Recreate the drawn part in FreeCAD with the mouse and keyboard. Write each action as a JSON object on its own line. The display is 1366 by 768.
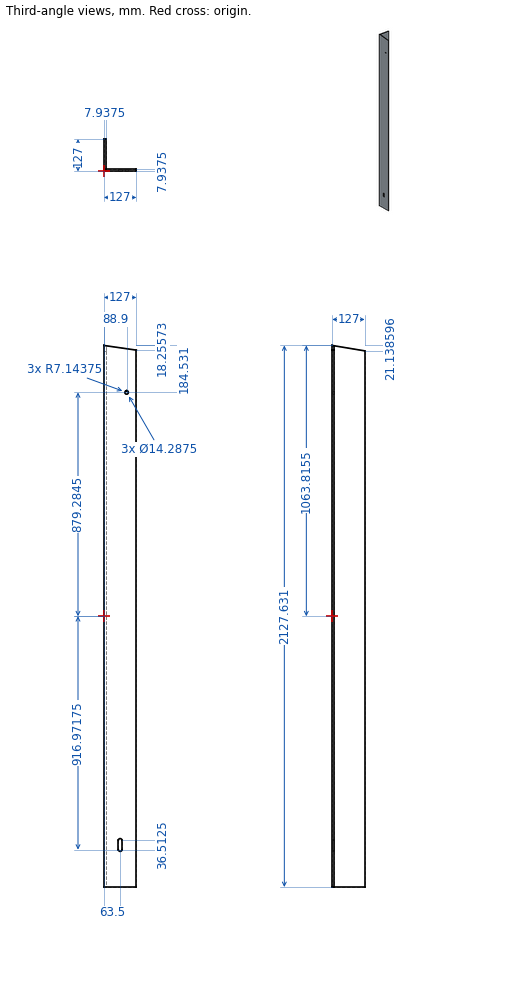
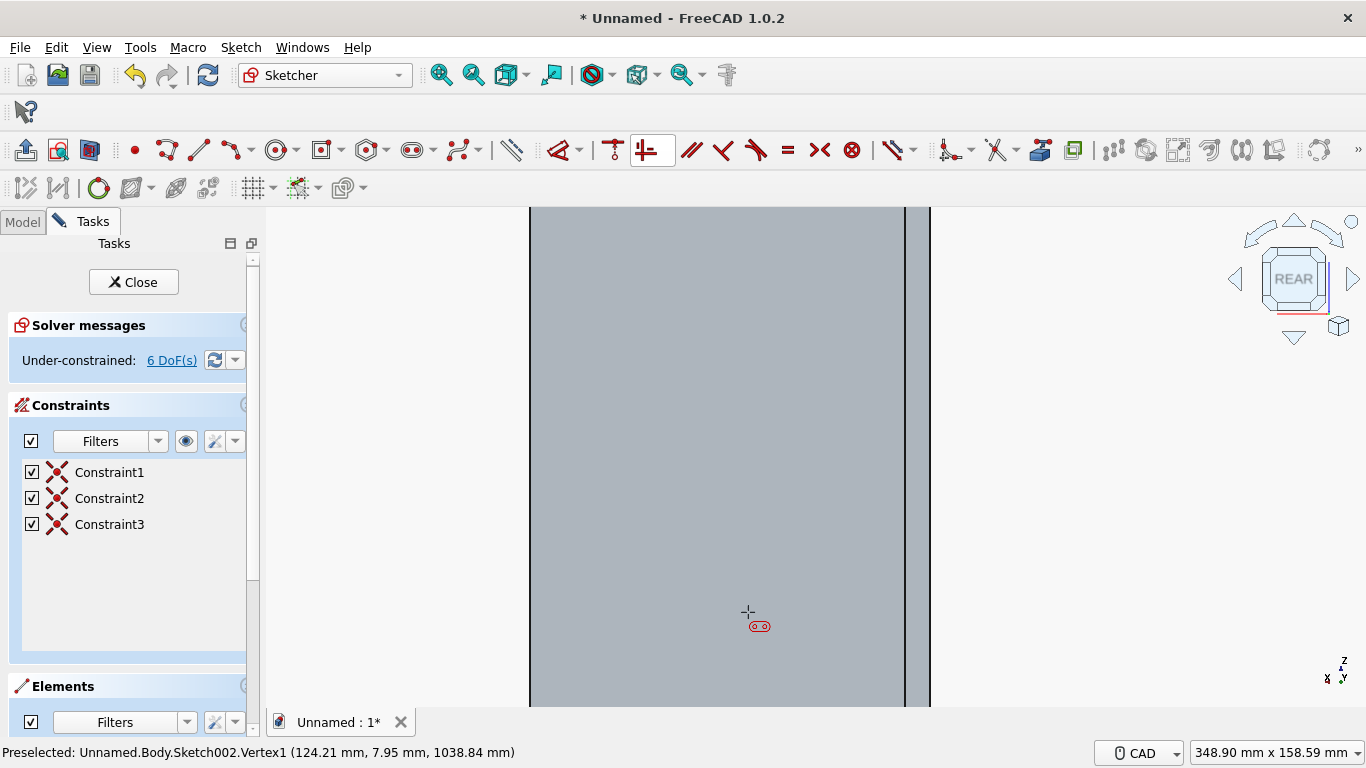
{"action": "scroll", "coordinate": [749, 649], "scroll_direction": "down", "scroll_amount": 15}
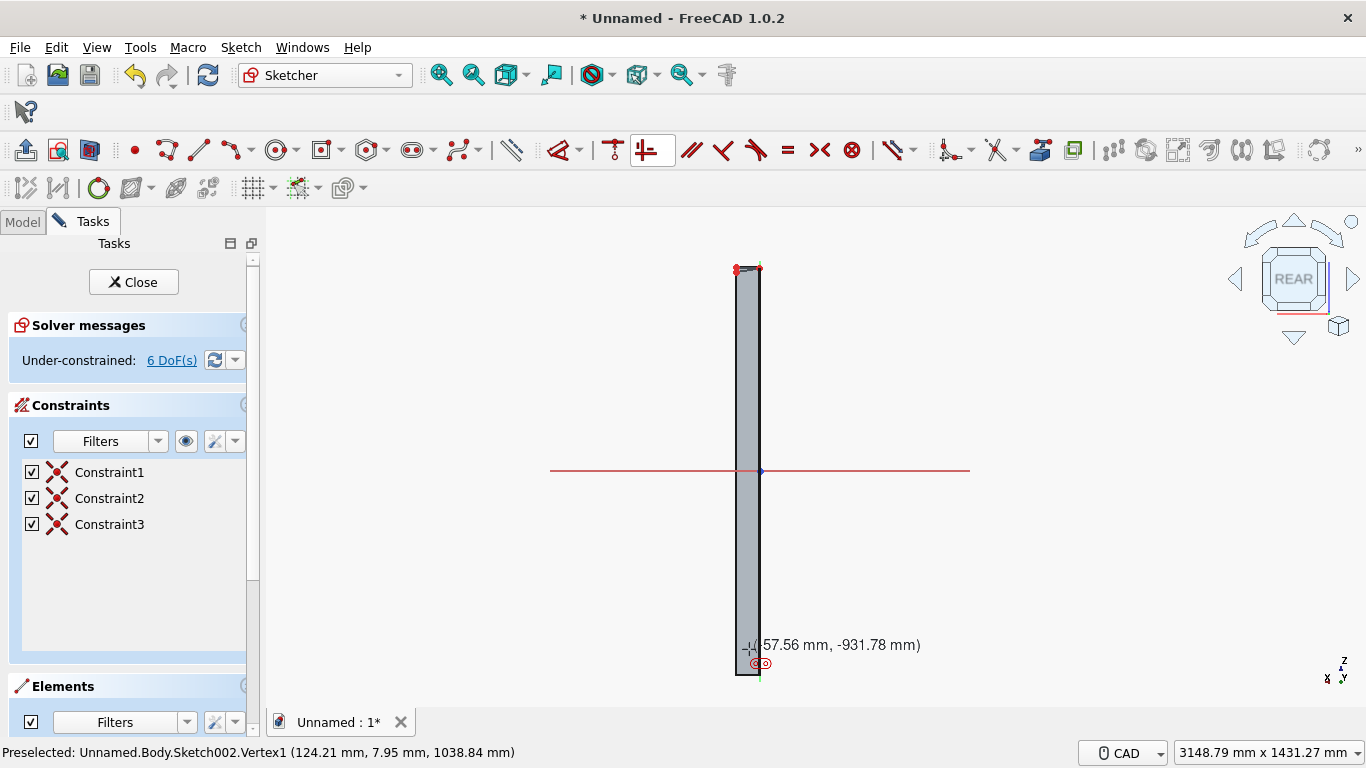
{"action": "scroll", "coordinate": [748, 647], "scroll_direction": "up", "scroll_amount": 2}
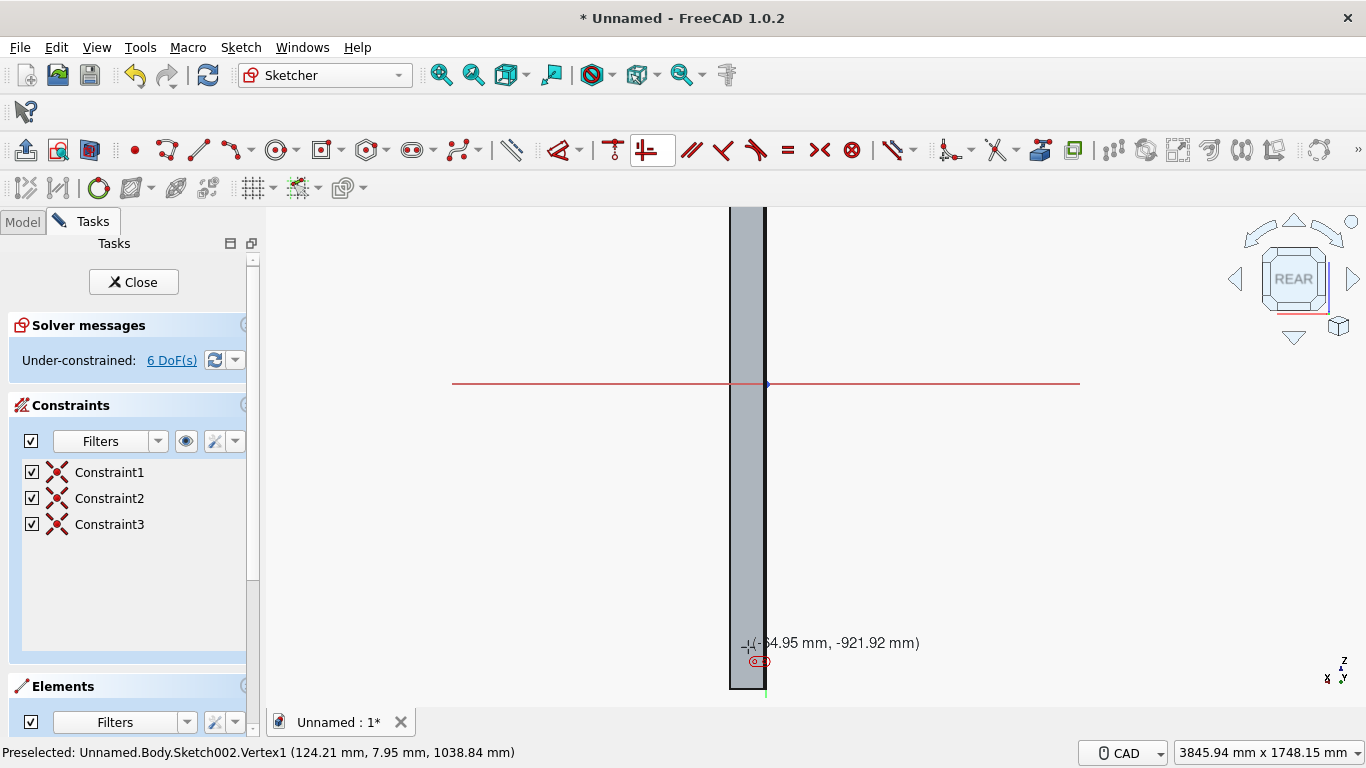
{"action": "left_click", "coordinate": [748, 647]}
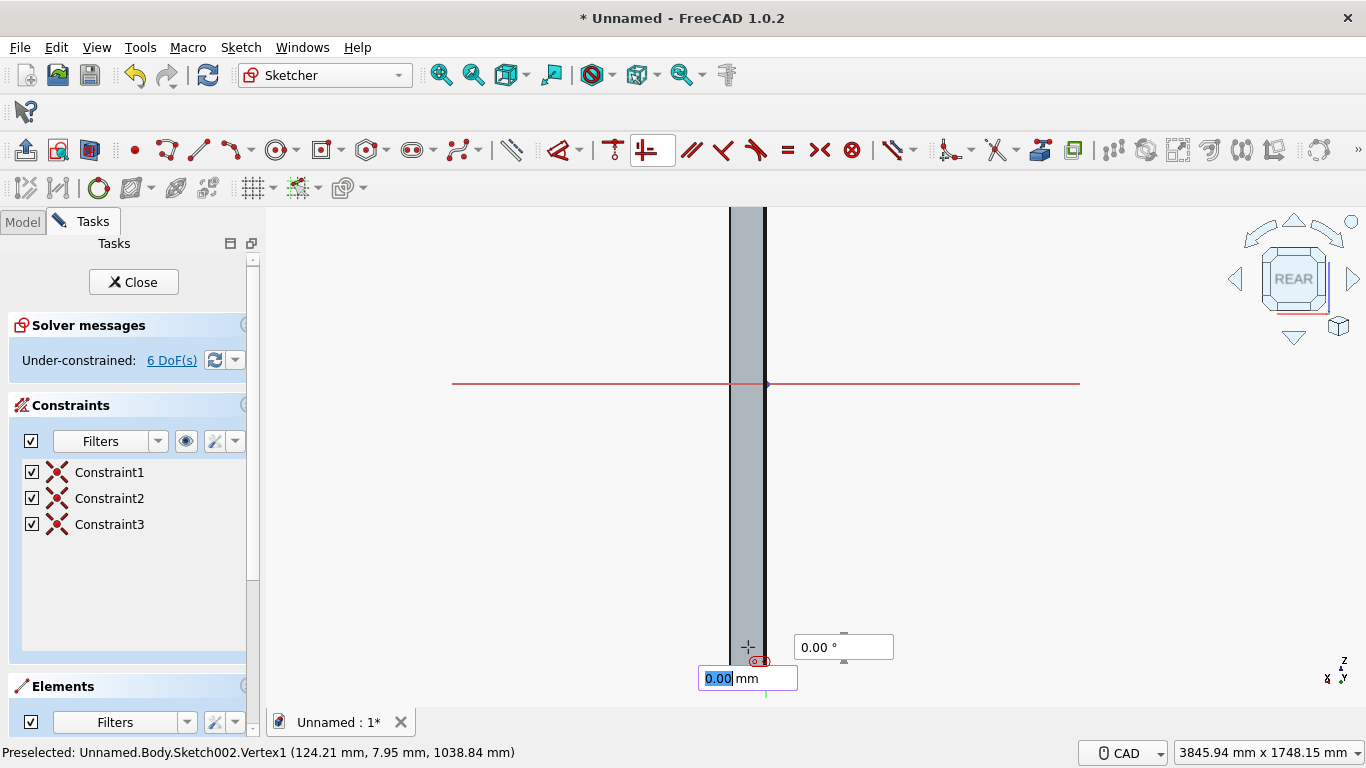
{"action": "scroll", "coordinate": [748, 636], "scroll_direction": "up", "scroll_amount": 3}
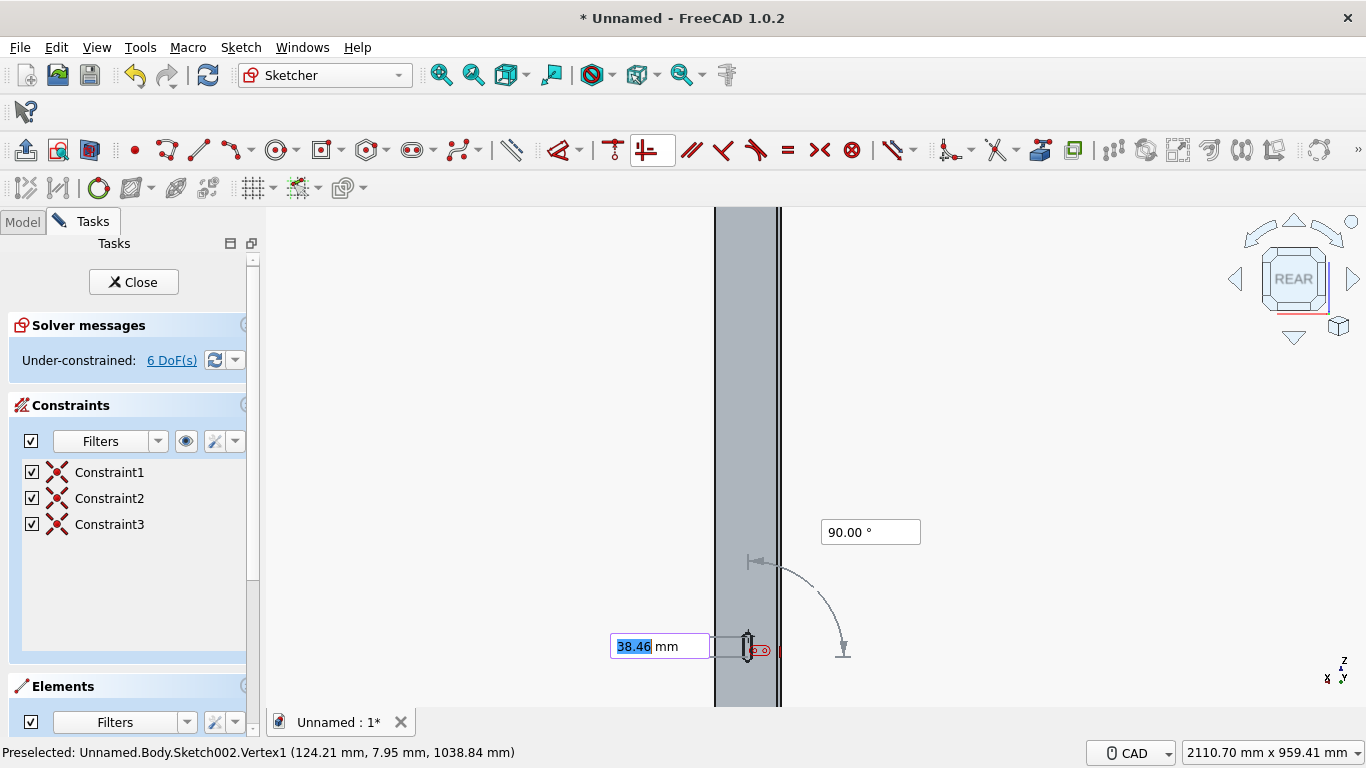
{"action": "left_click", "coordinate": [748, 636]}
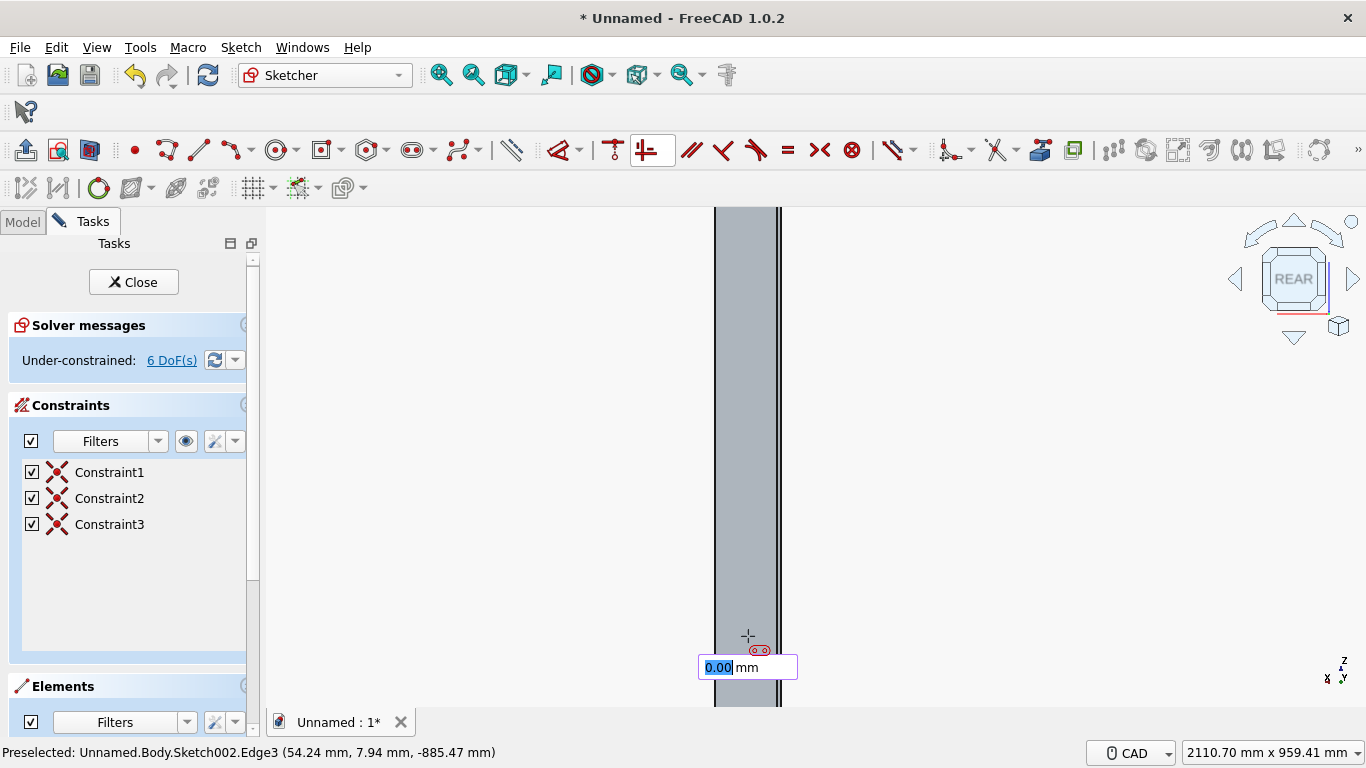
{"action": "scroll", "coordinate": [744, 645], "scroll_direction": "up", "scroll_amount": 8}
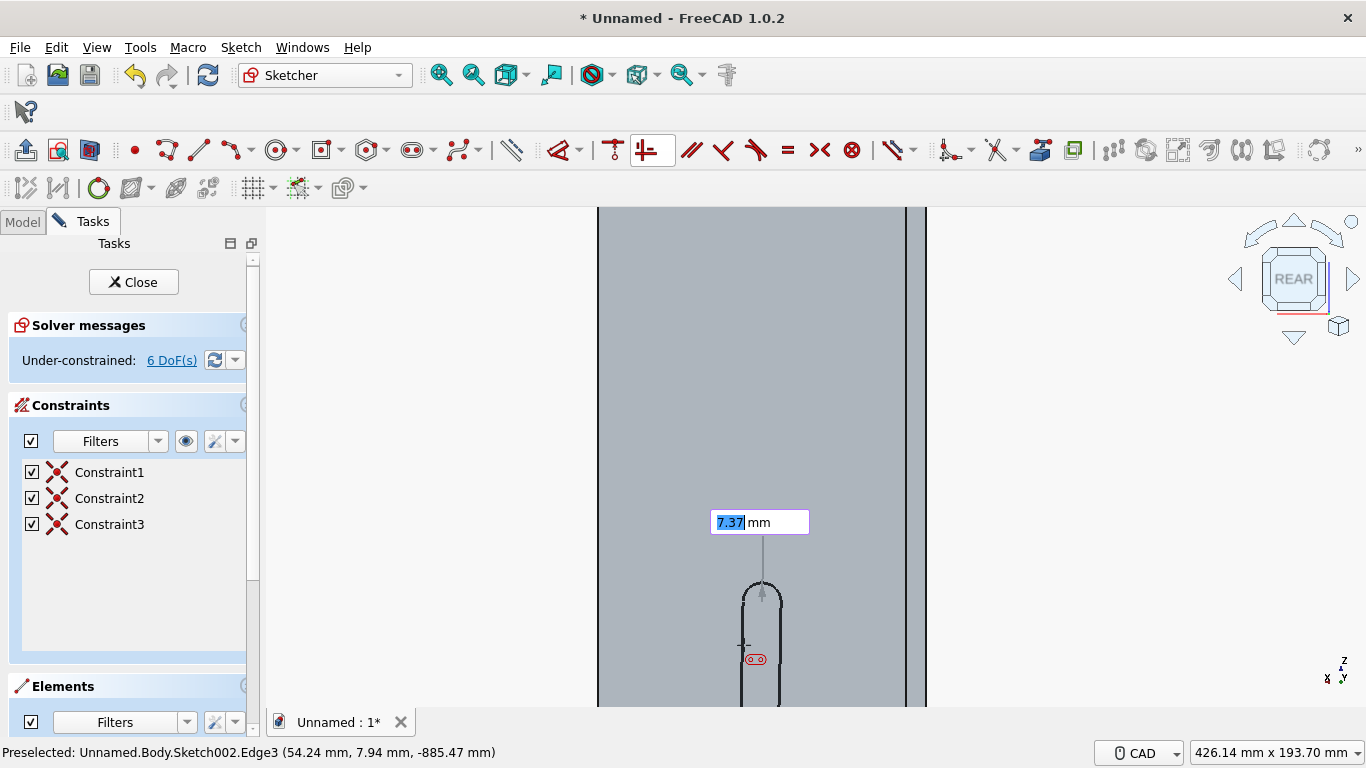
{"action": "left_click", "coordinate": [744, 642]}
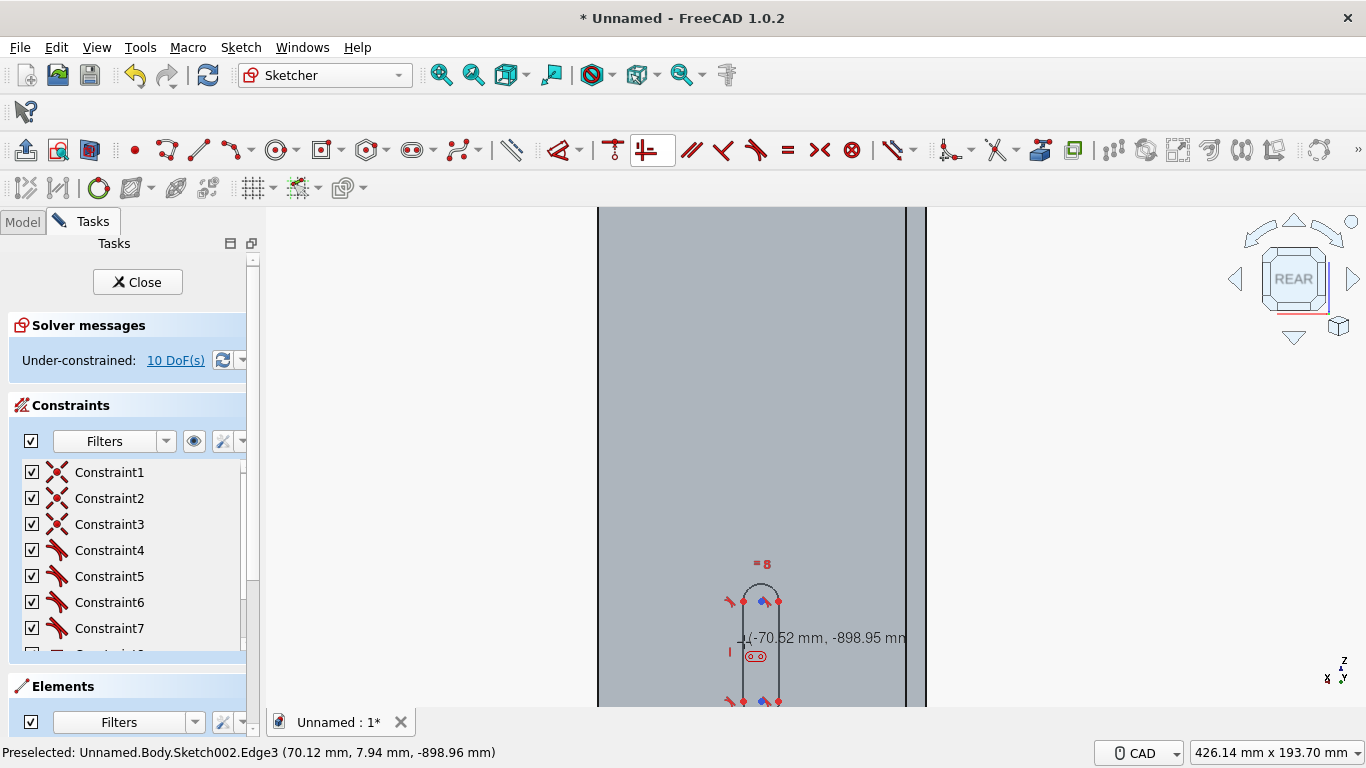
{"action": "key", "text": "g c"}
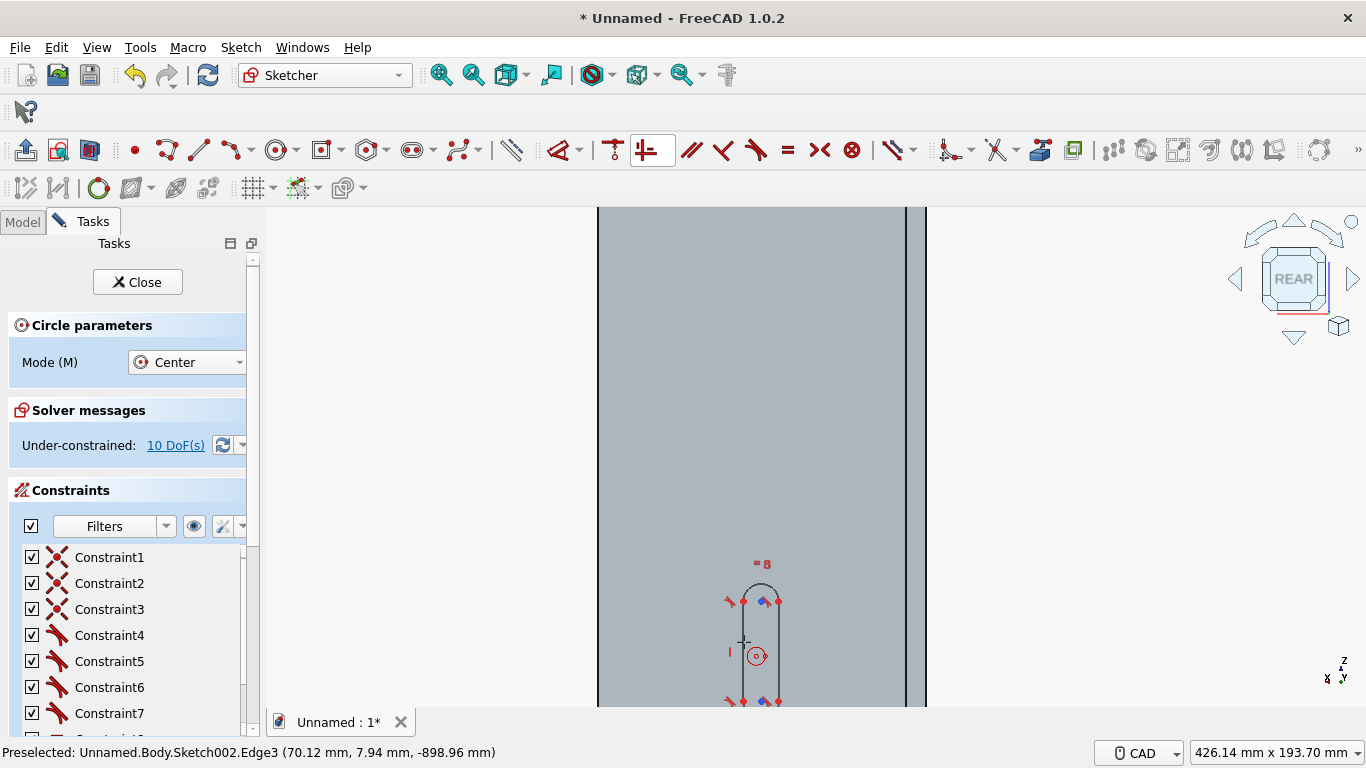
{"action": "scroll", "coordinate": [747, 607], "scroll_direction": "down", "scroll_amount": 14}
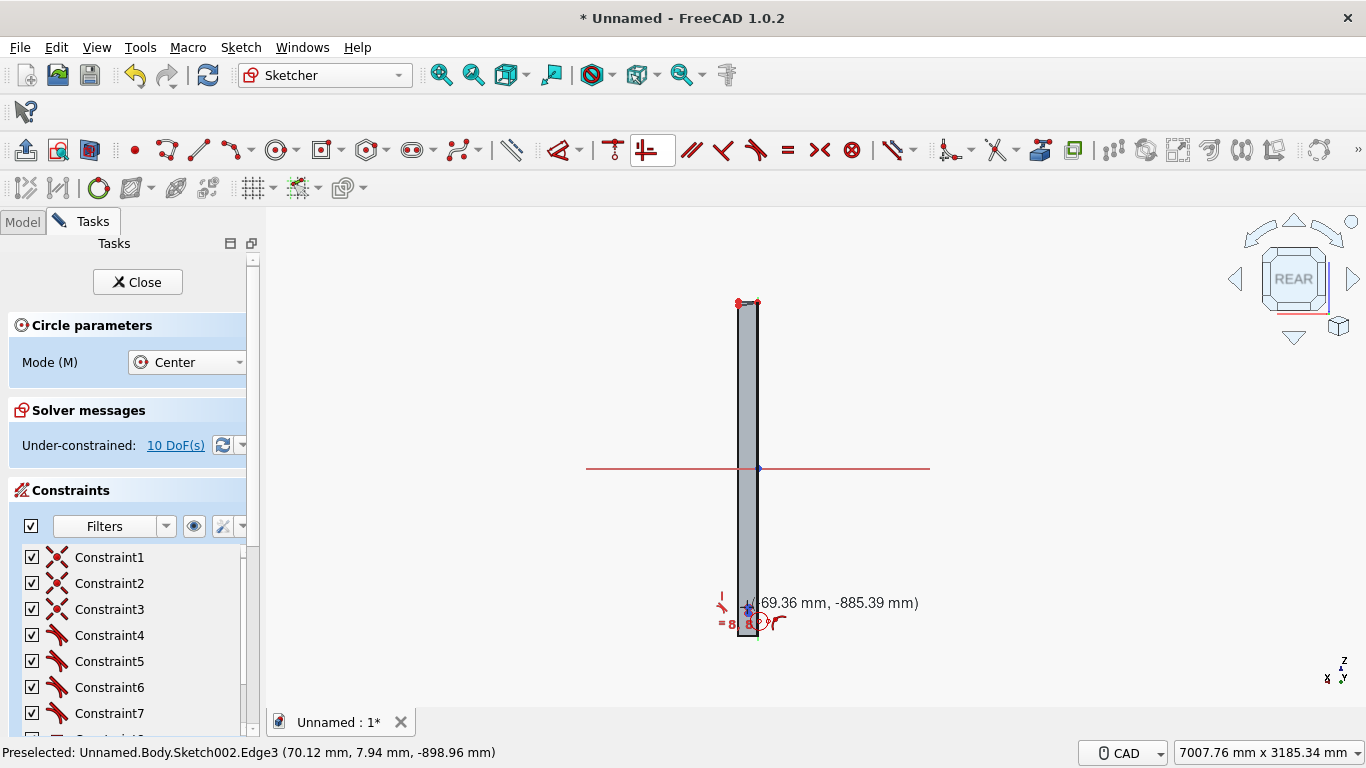
{"action": "scroll", "coordinate": [744, 331], "scroll_direction": "up", "scroll_amount": 16}